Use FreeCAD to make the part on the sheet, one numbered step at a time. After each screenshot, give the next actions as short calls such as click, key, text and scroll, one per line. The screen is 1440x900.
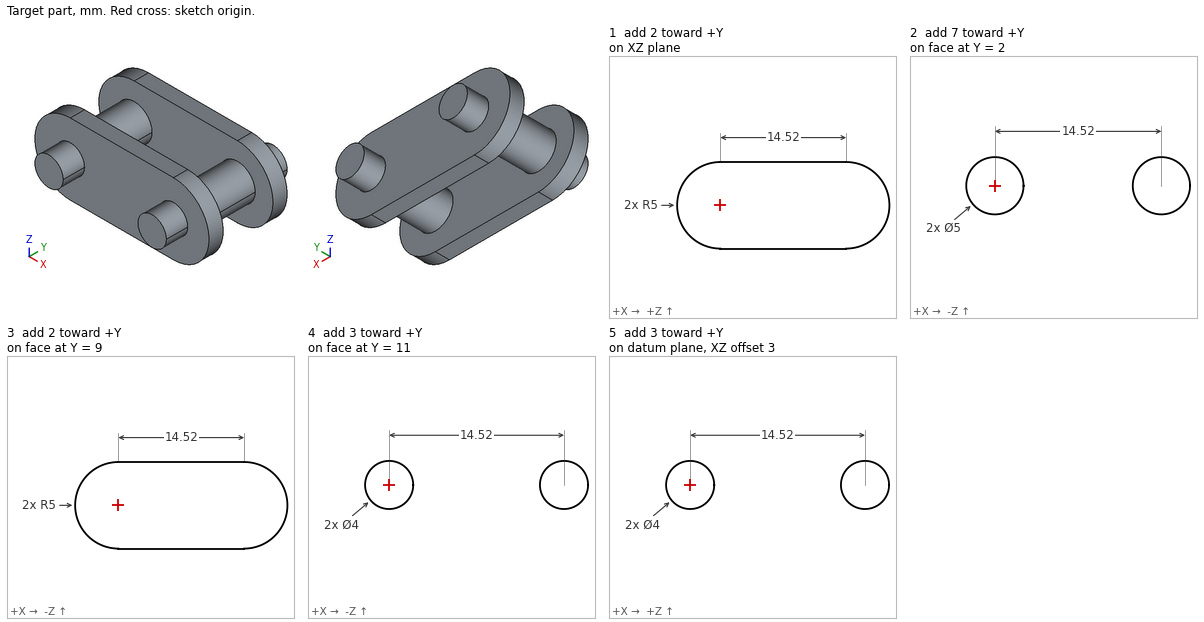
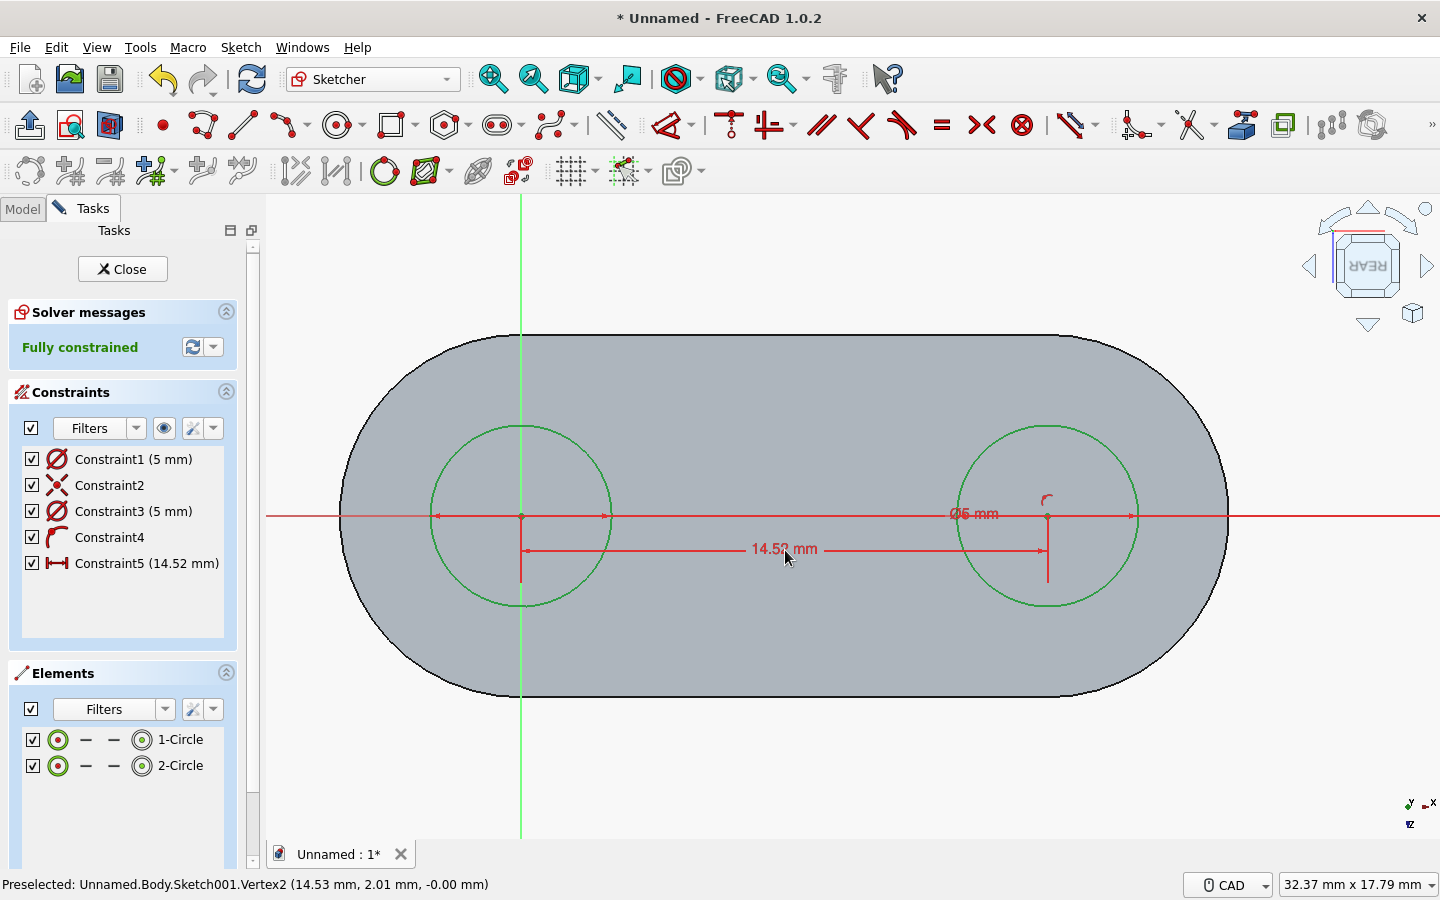
click(123, 269)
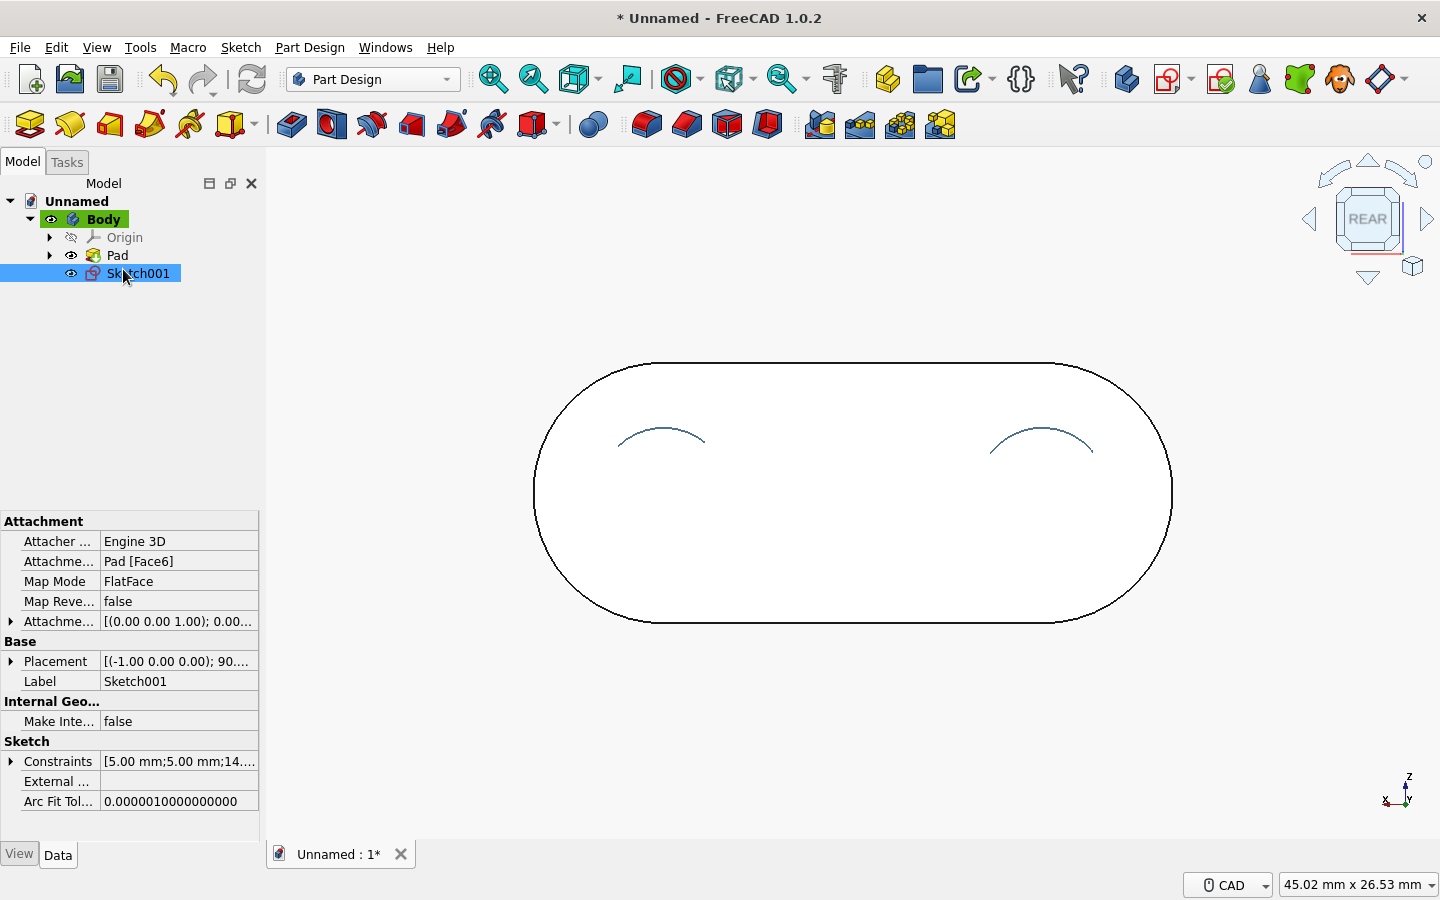
click(30, 124)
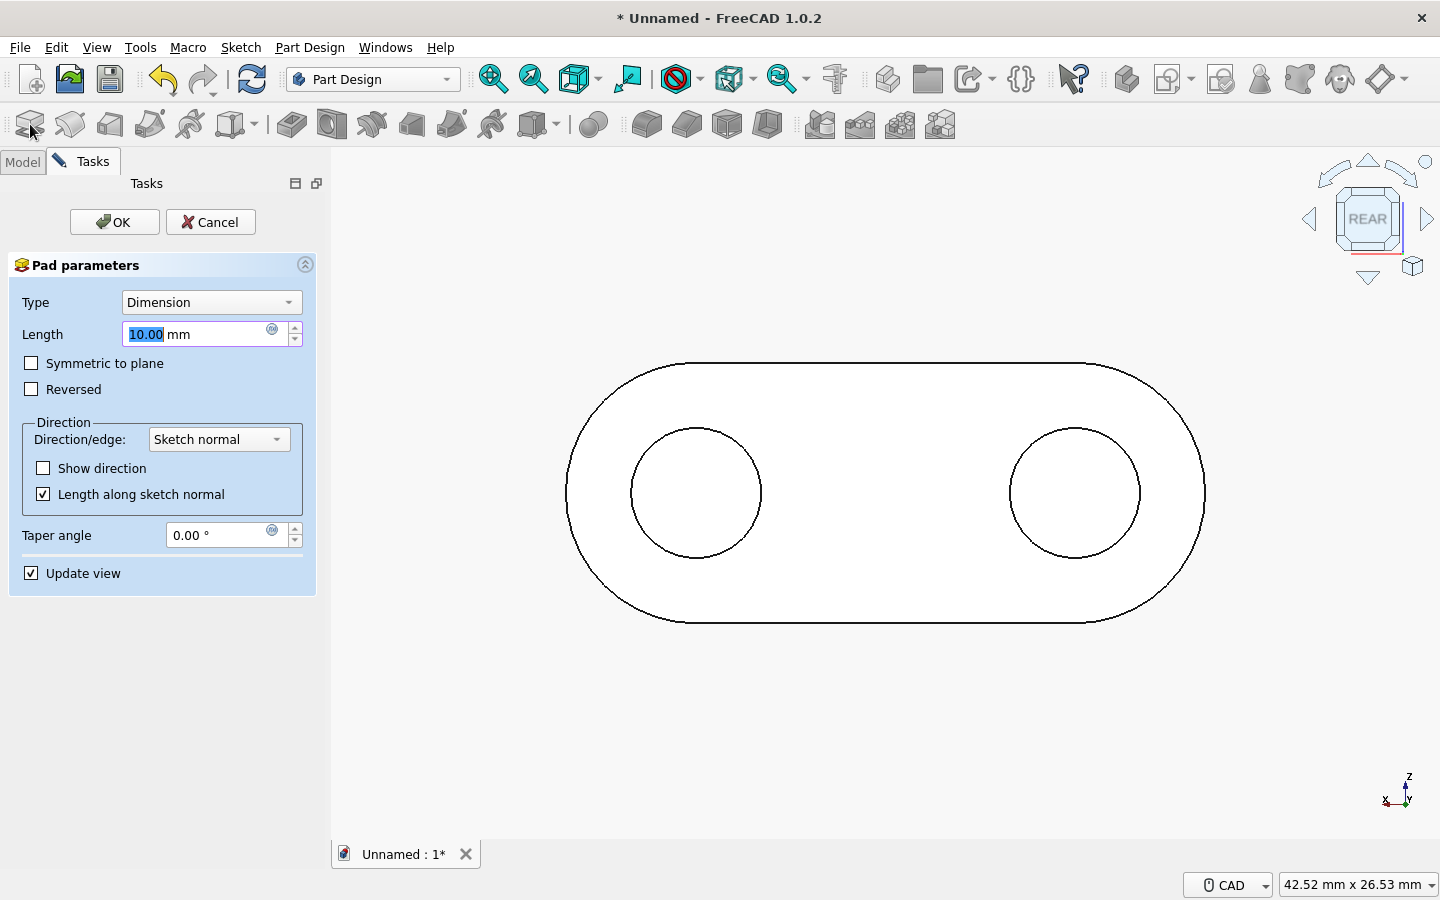
text(7)
key(Tab)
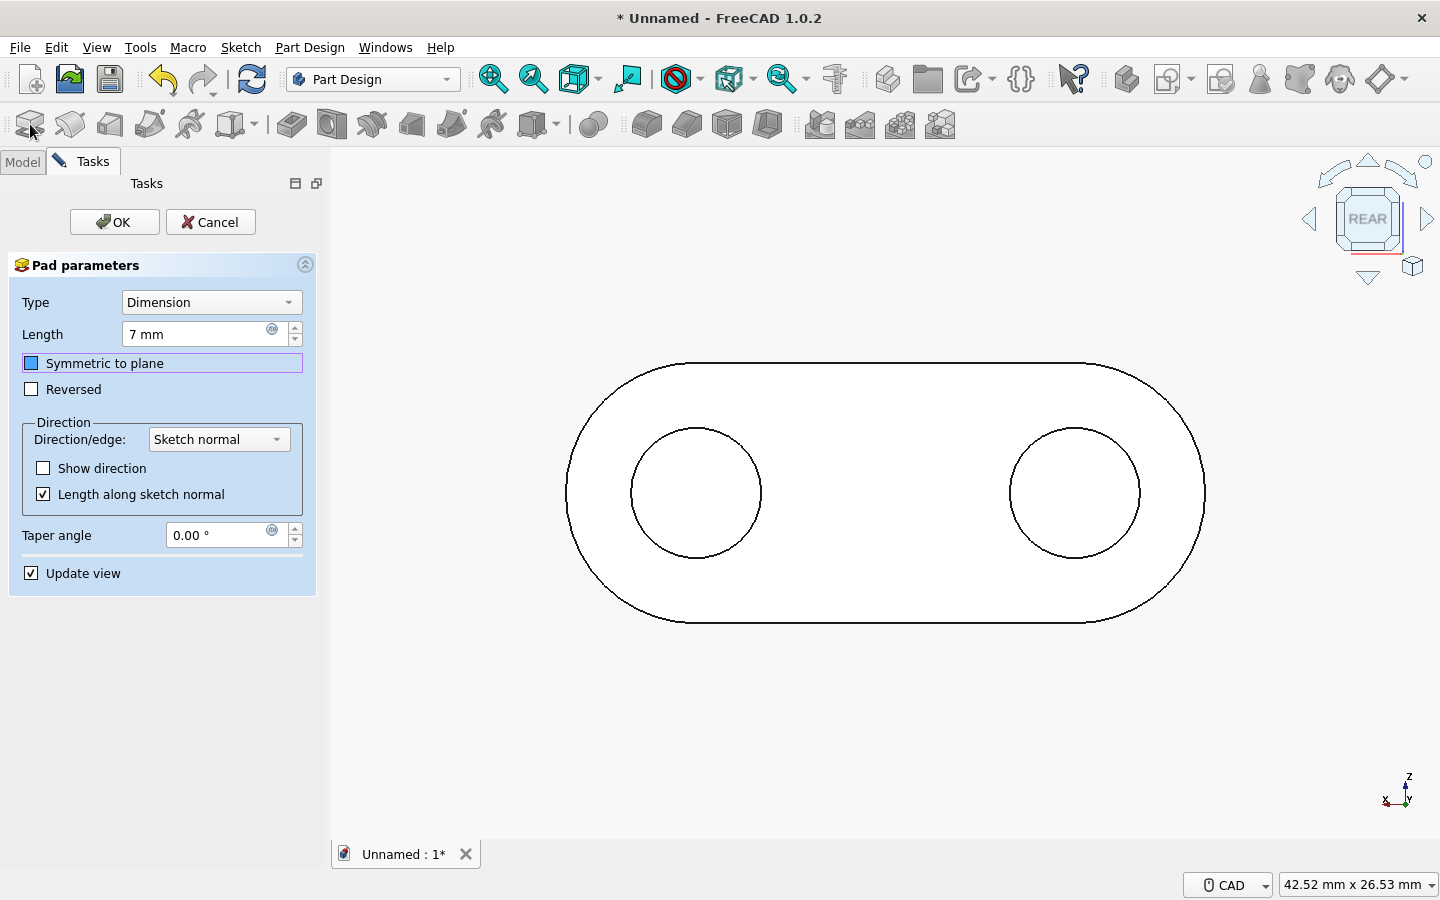
click(115, 222)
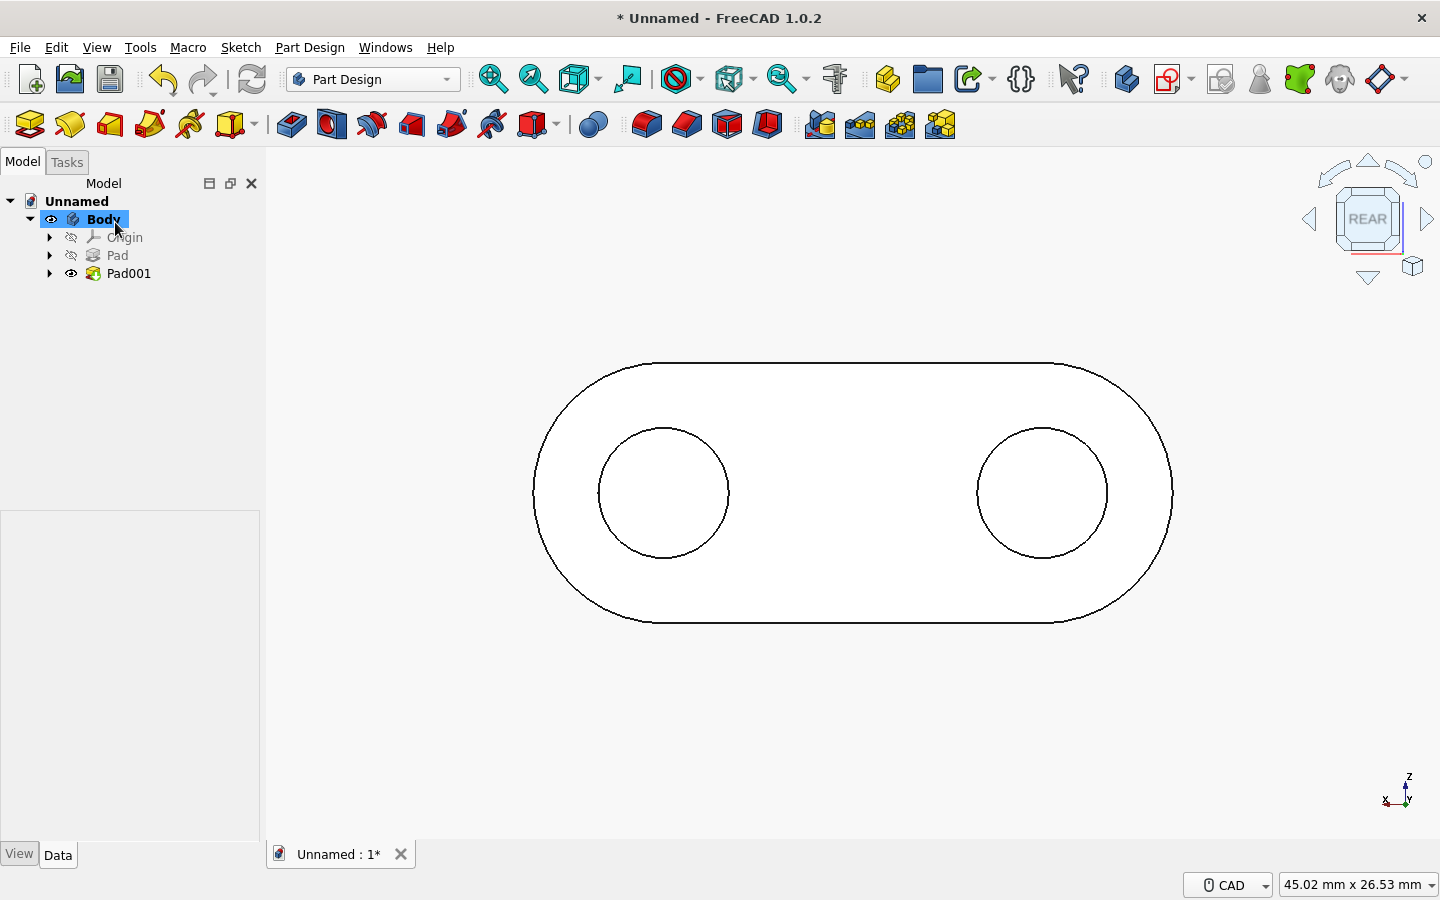
click(1042, 492)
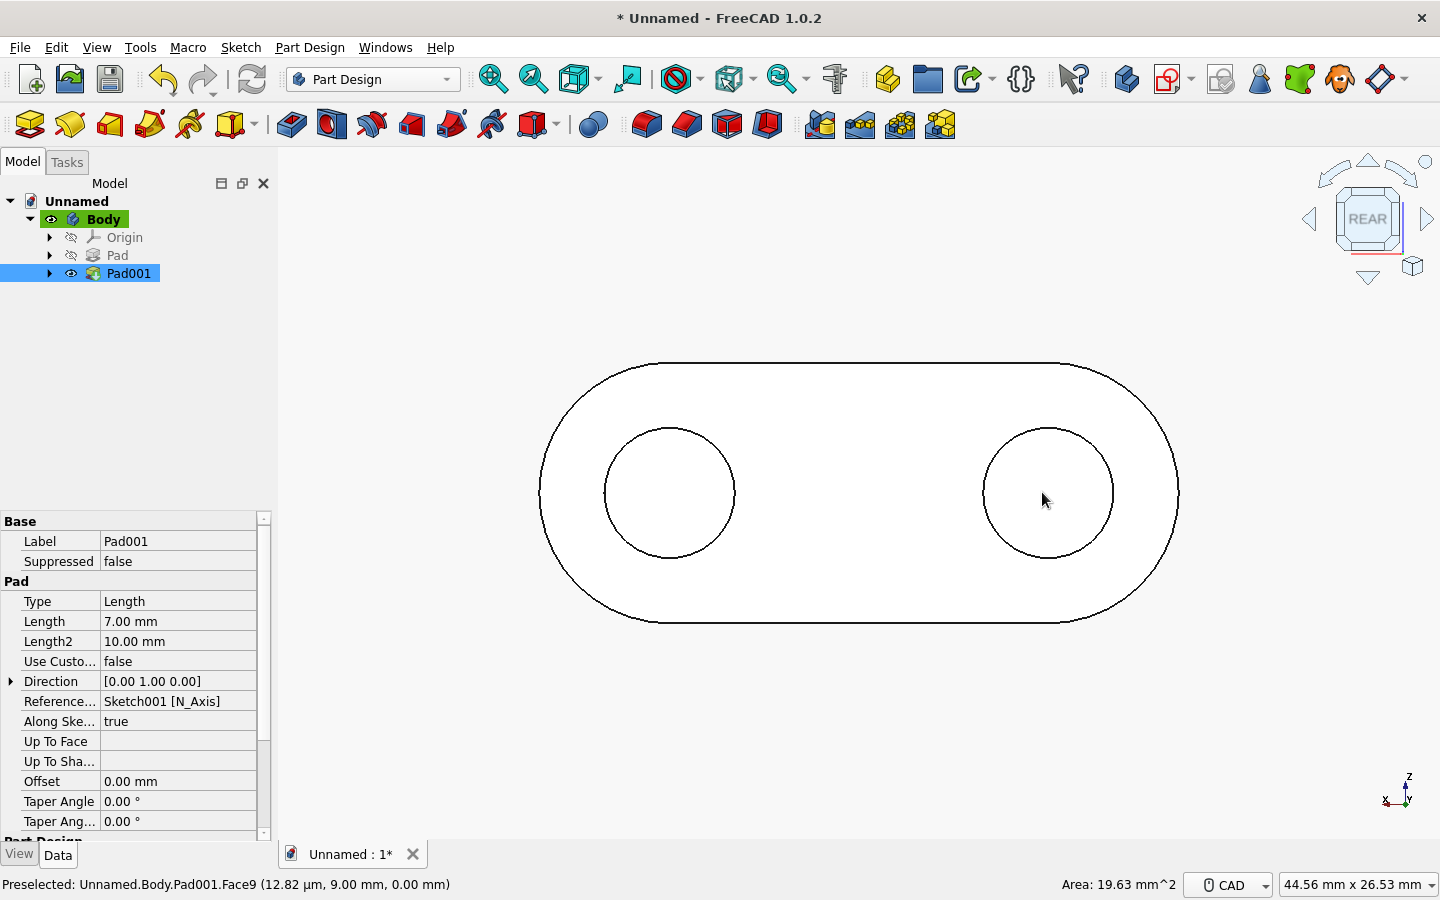
click(1168, 80)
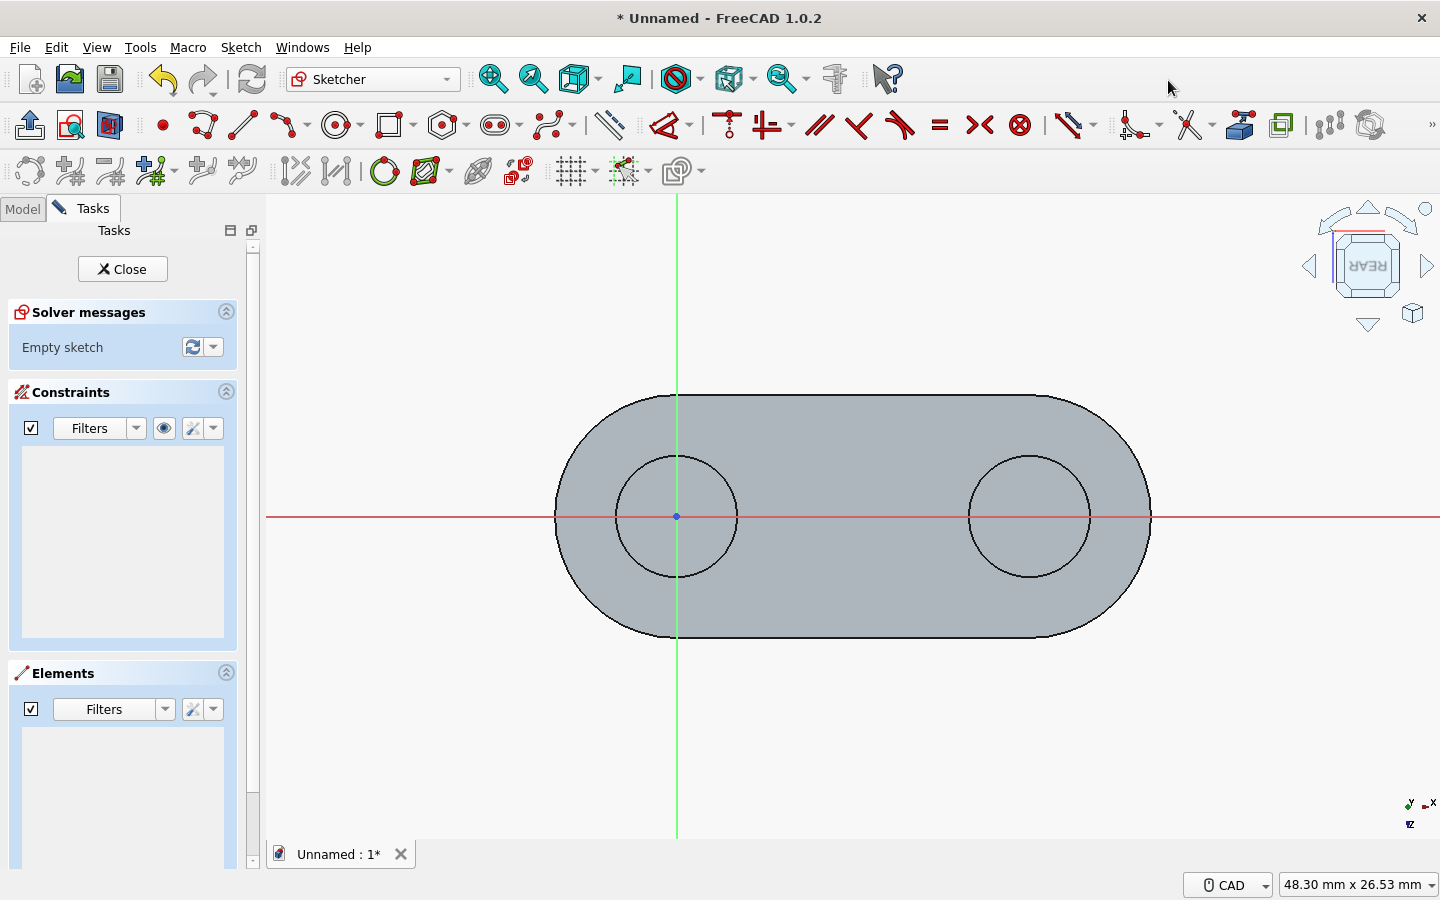
key(g)
key(s)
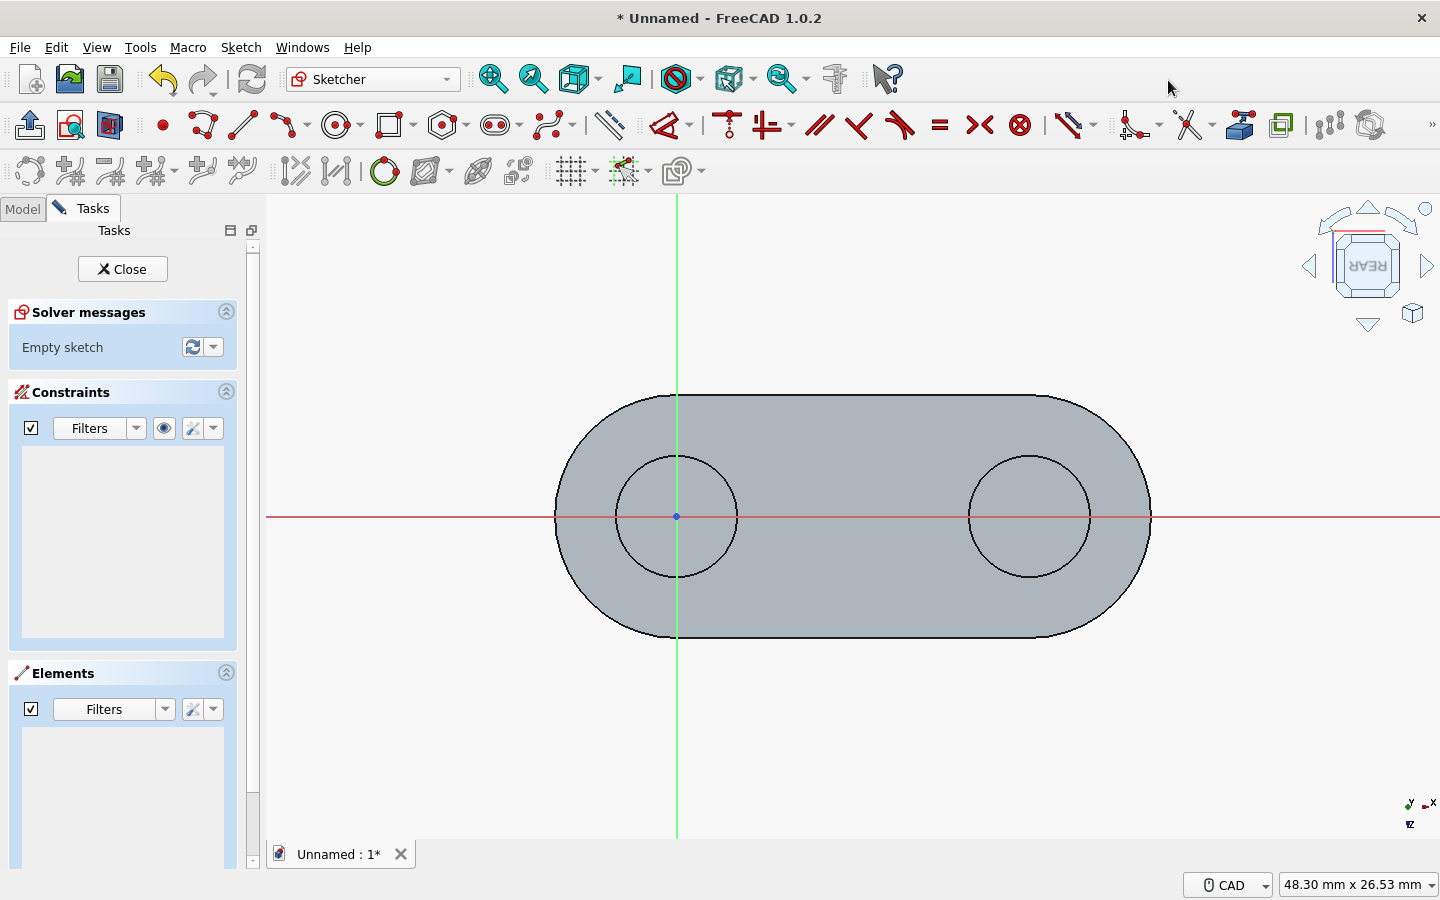
click(677, 516)